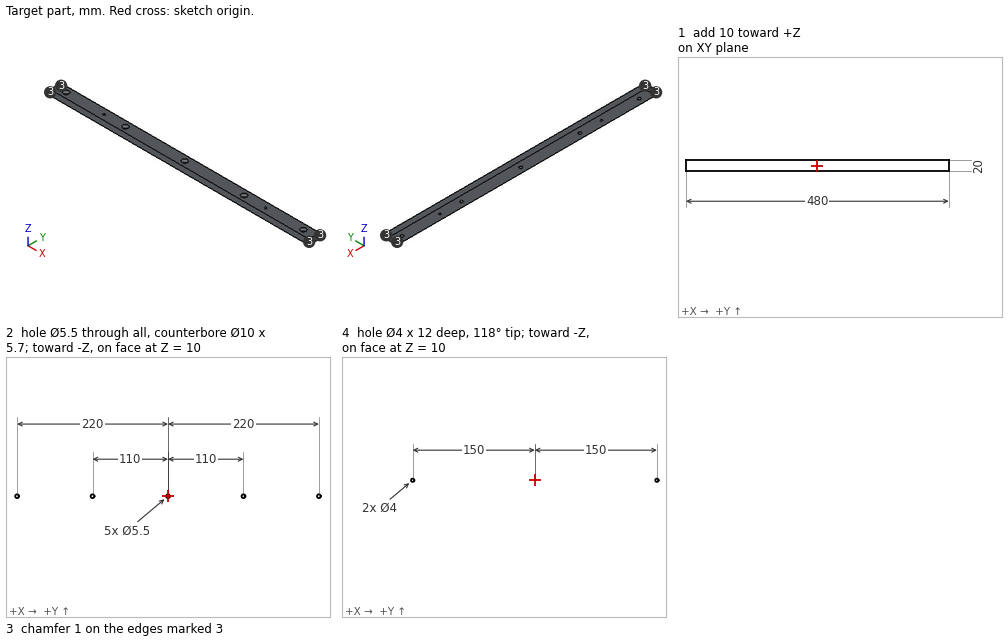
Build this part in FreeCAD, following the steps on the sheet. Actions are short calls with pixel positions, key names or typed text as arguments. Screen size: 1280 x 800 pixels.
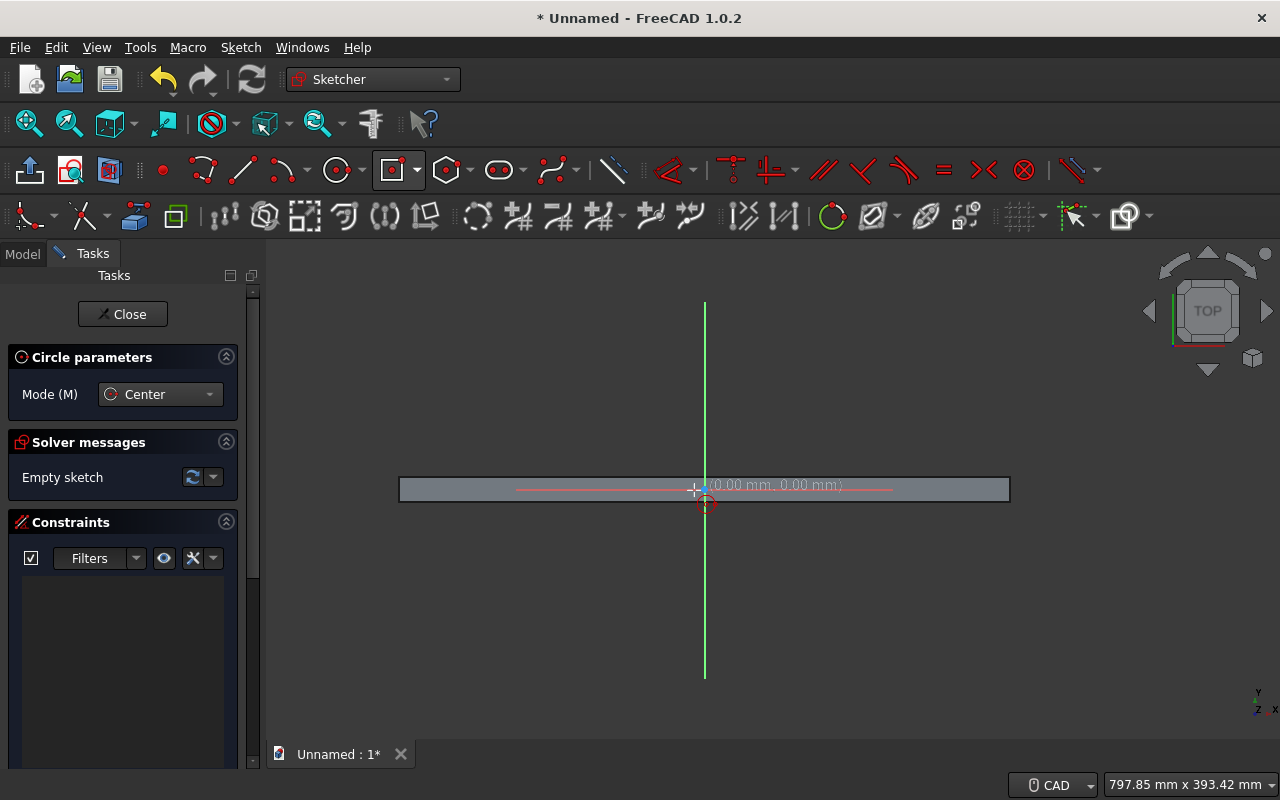
click(705, 490)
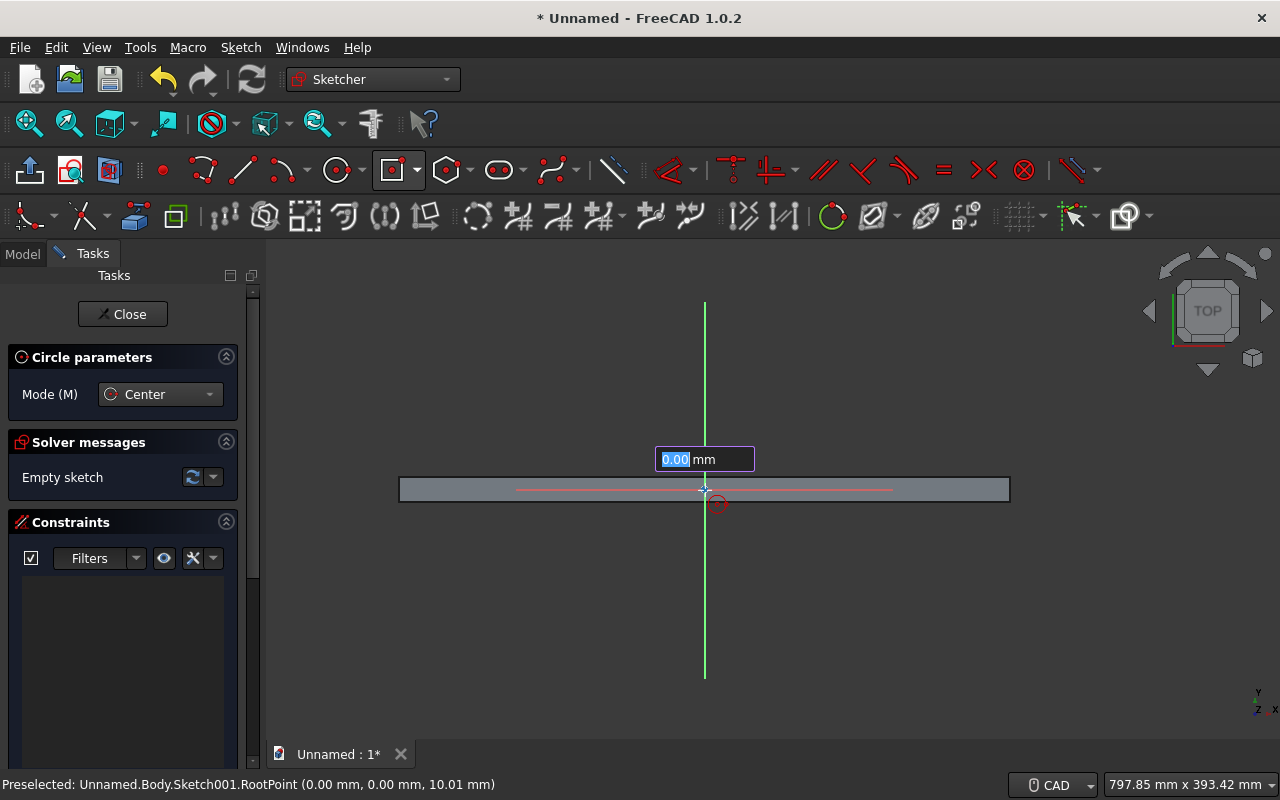
scroll(707, 487, up, 10)
move(704, 486)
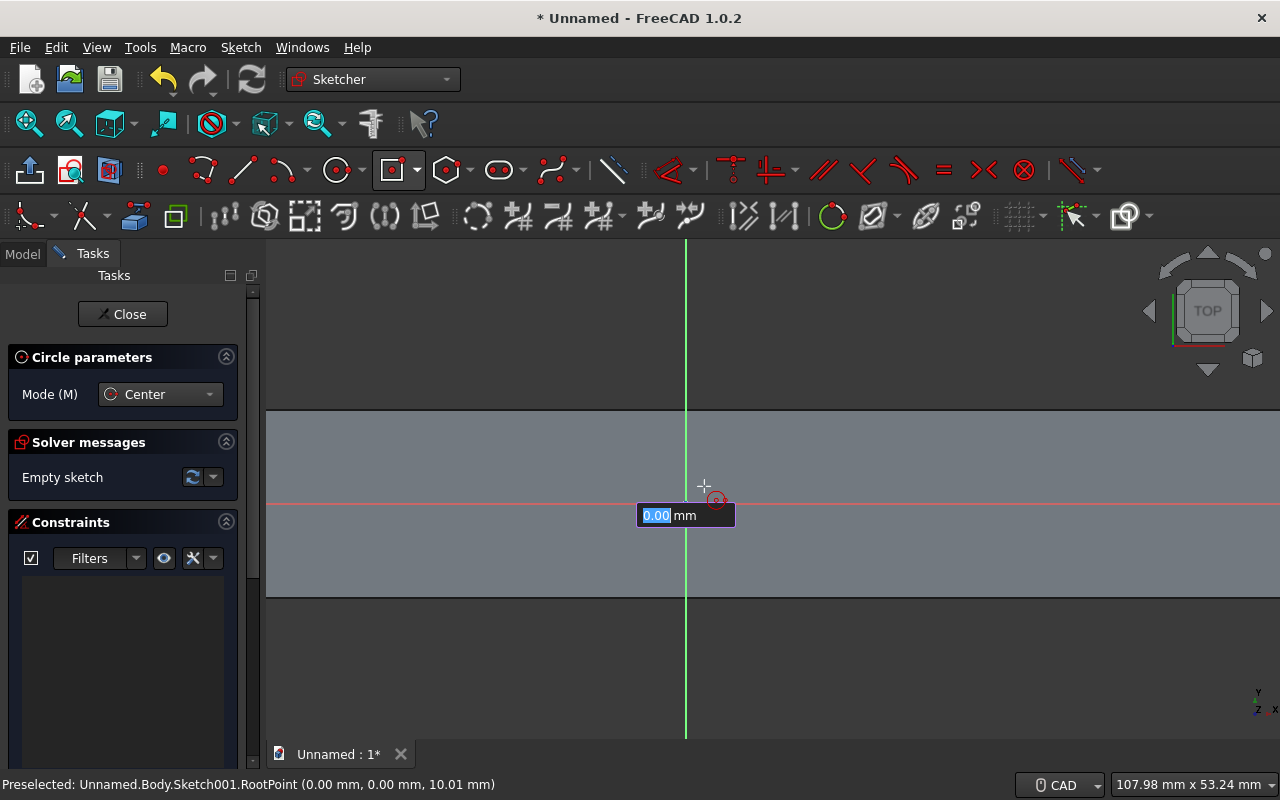
text(5.5)
key(Return)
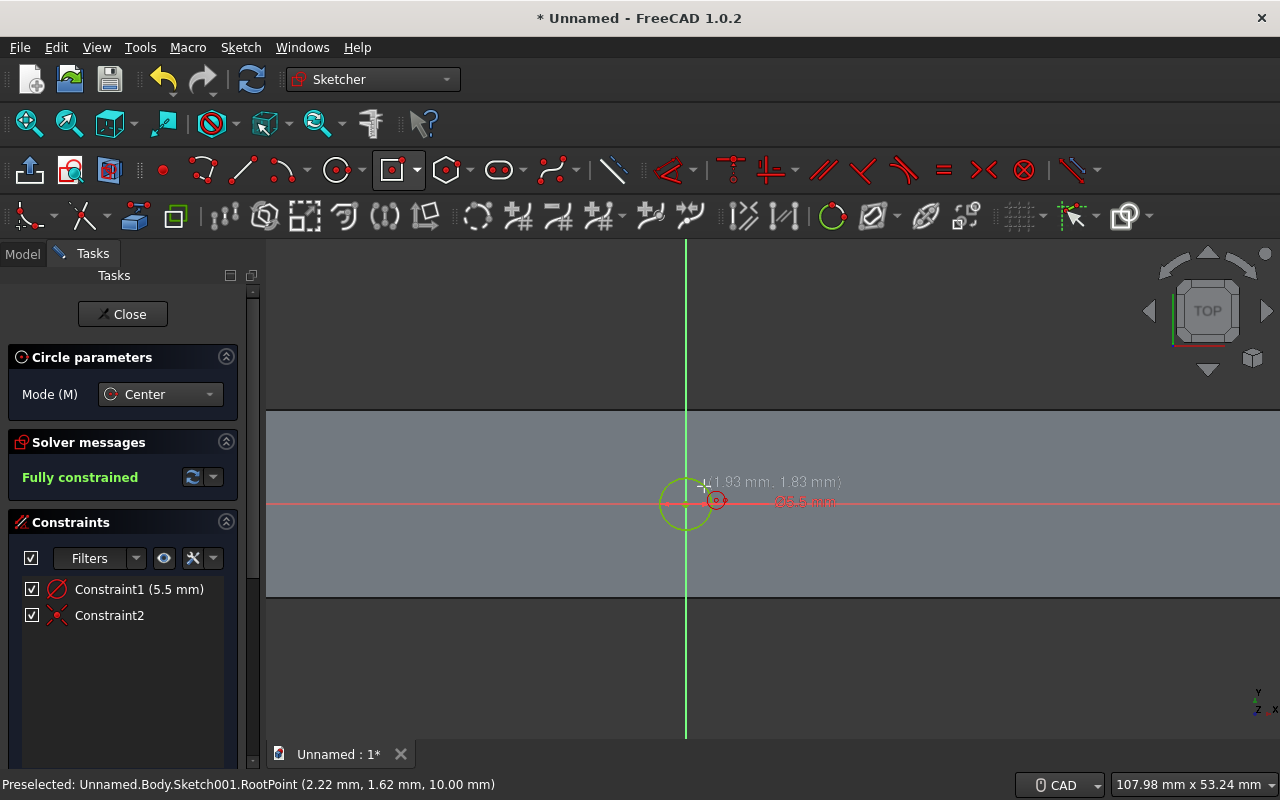
scroll(707, 487, down, 10)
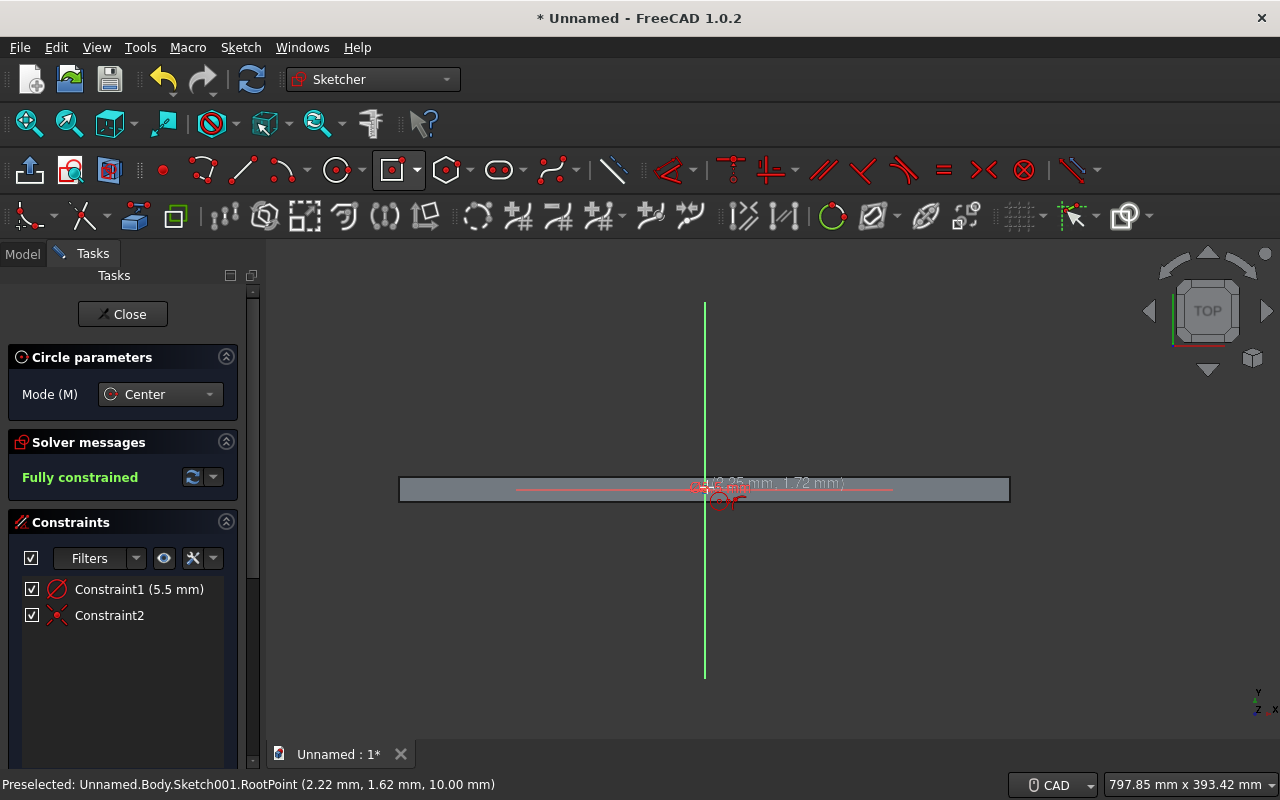
scroll(565, 490, up, 10)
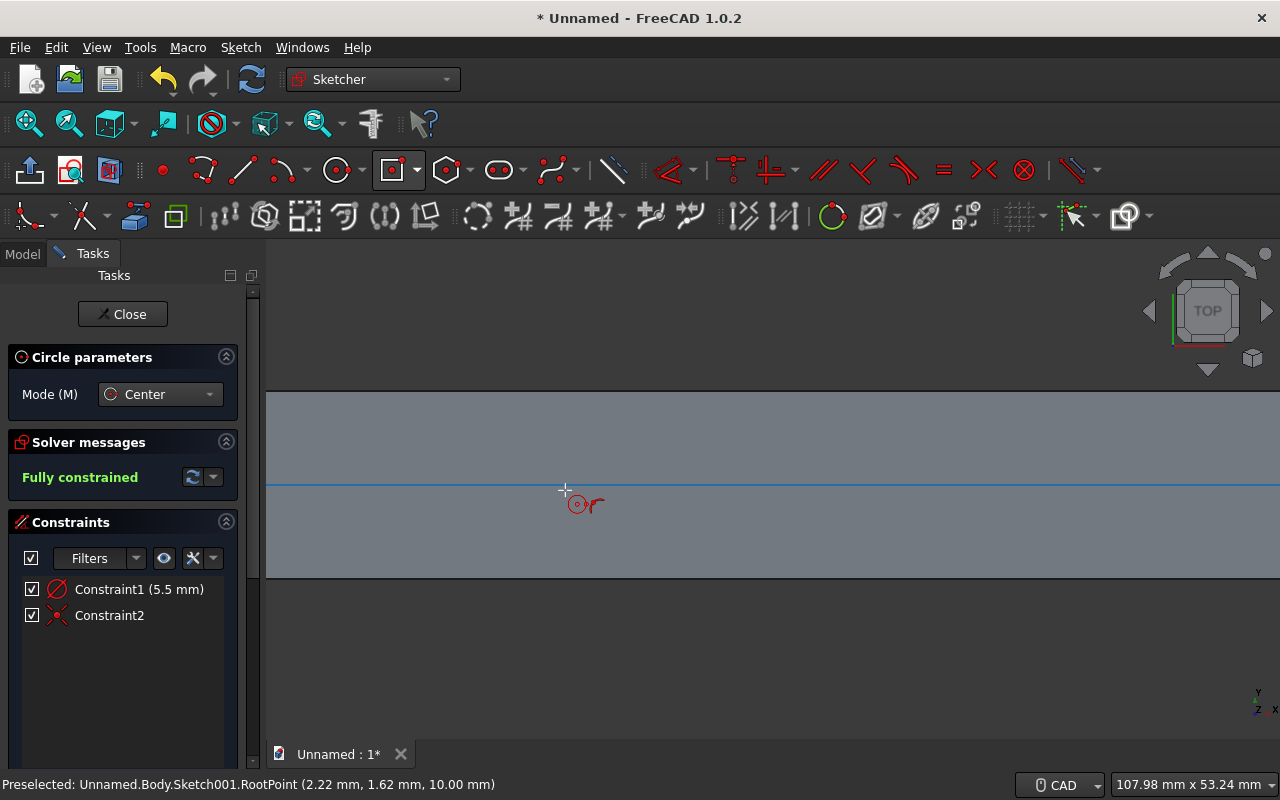
scroll(565, 490, down, 10)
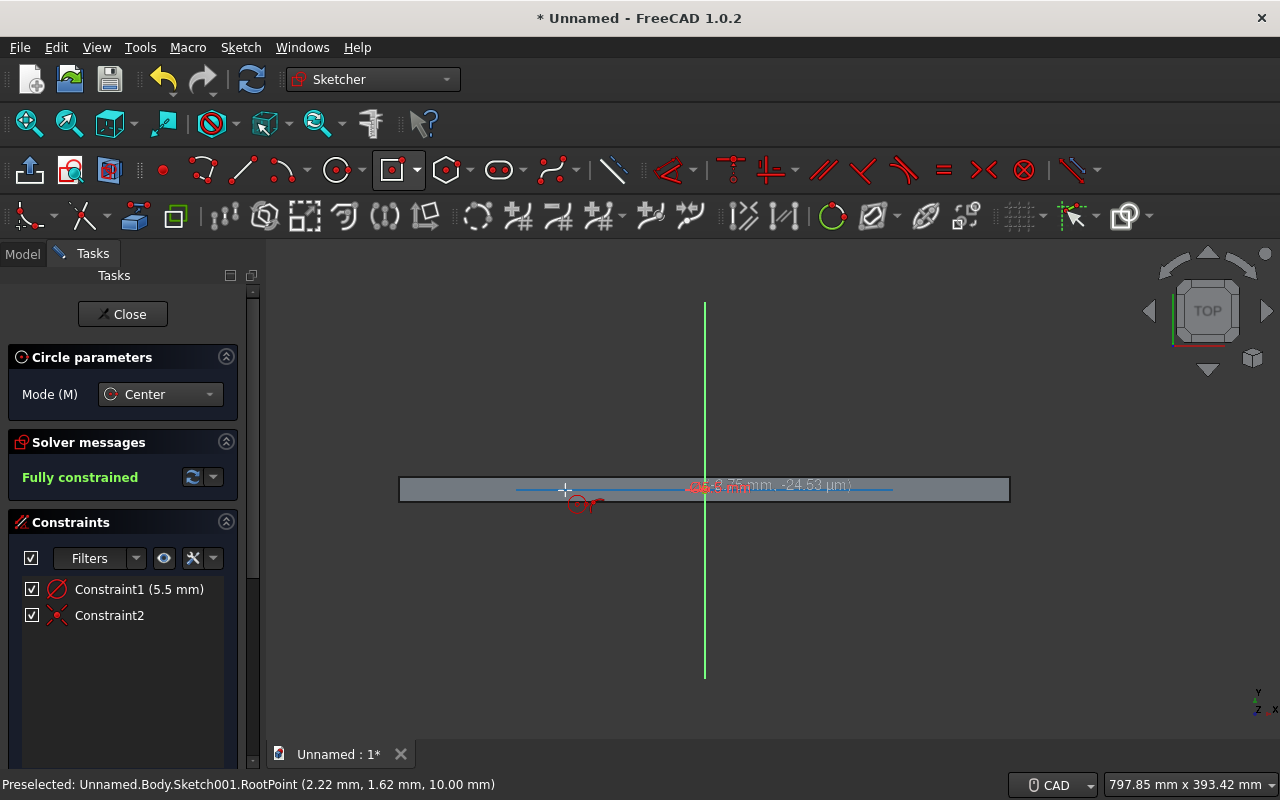
click(565, 490)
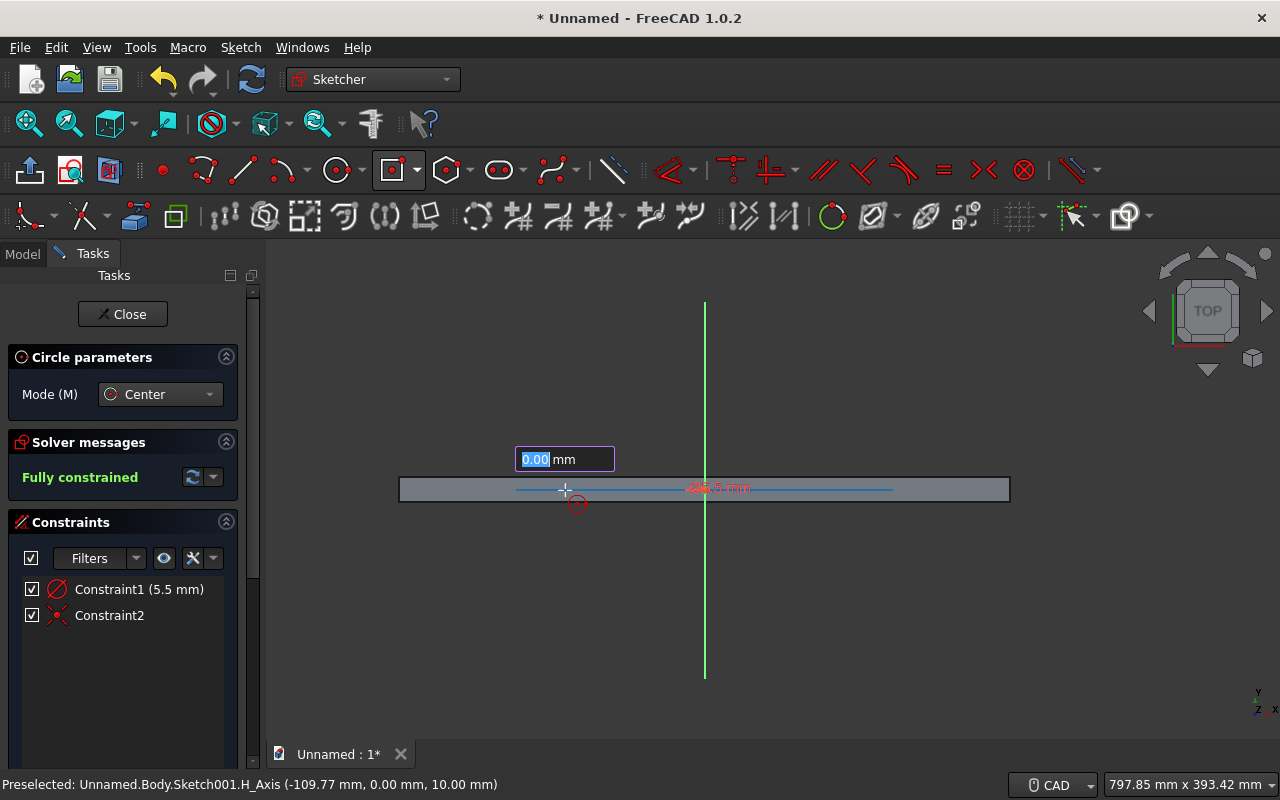
scroll(566, 486, up, 8)
move(564, 486)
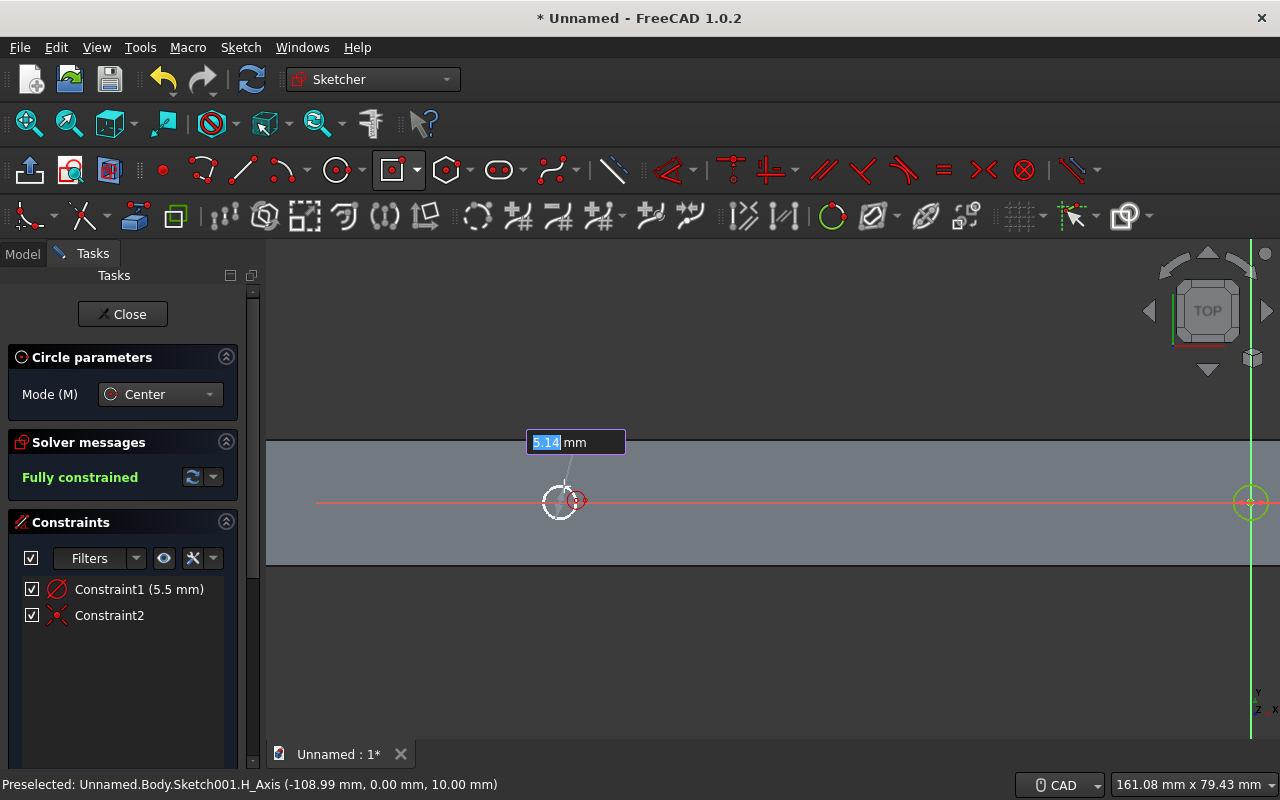
text(5.5)
key(Return)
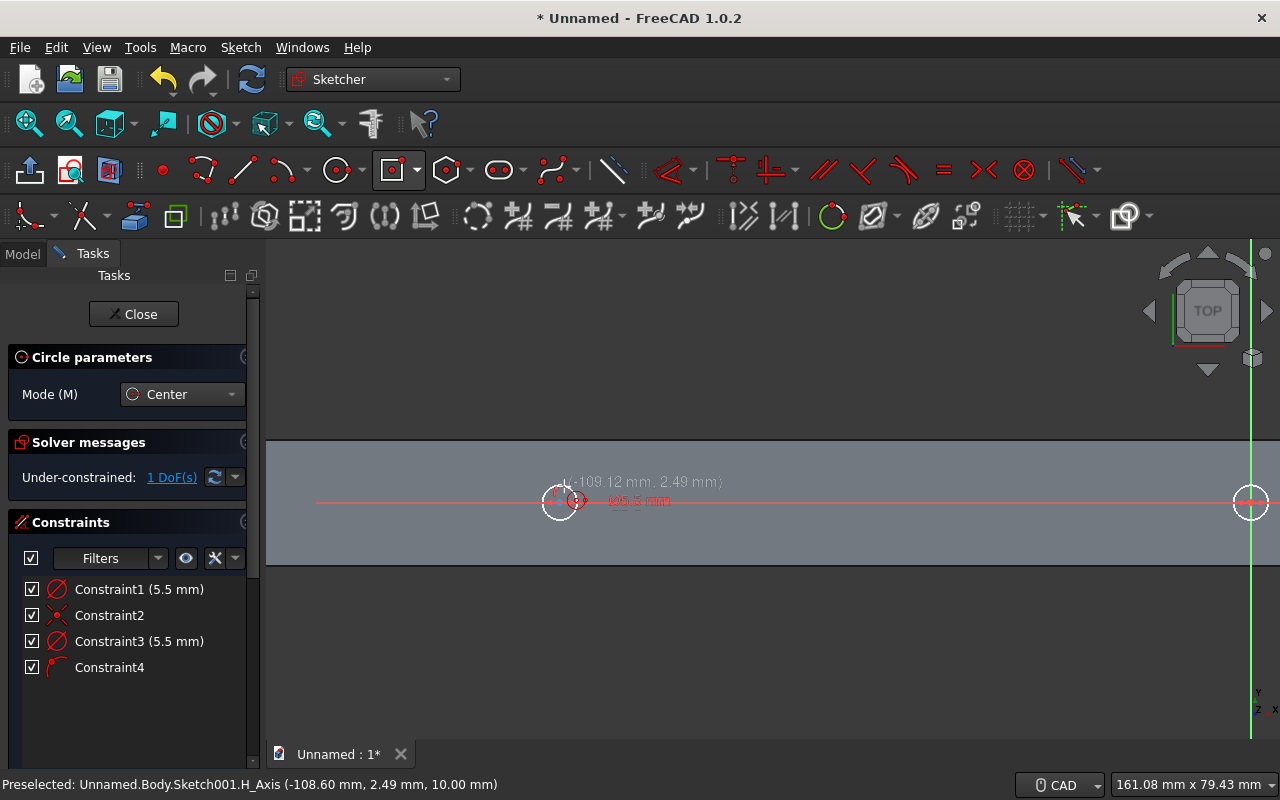
scroll(566, 486, down, 8)